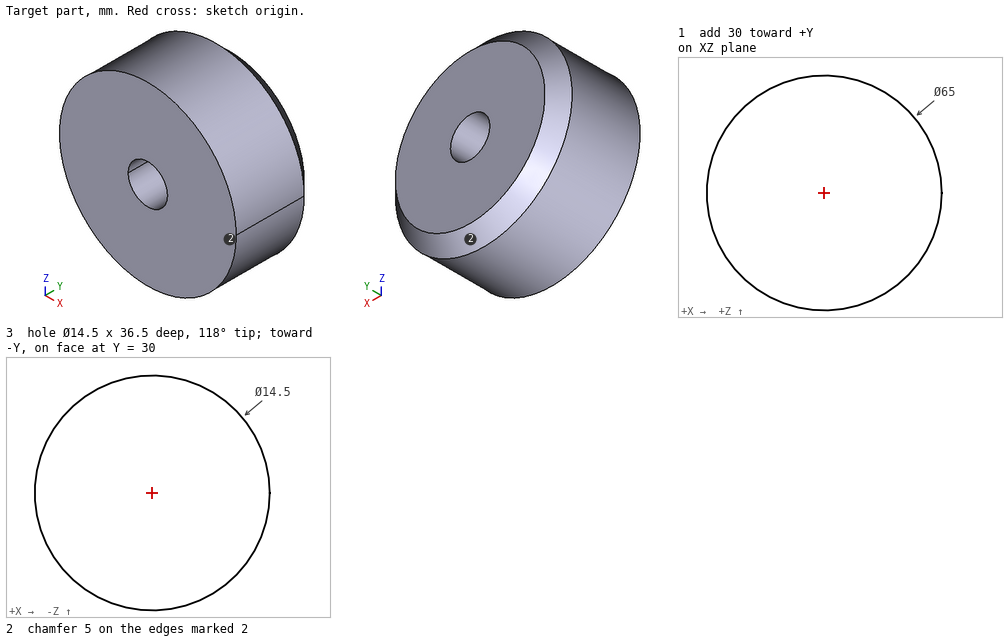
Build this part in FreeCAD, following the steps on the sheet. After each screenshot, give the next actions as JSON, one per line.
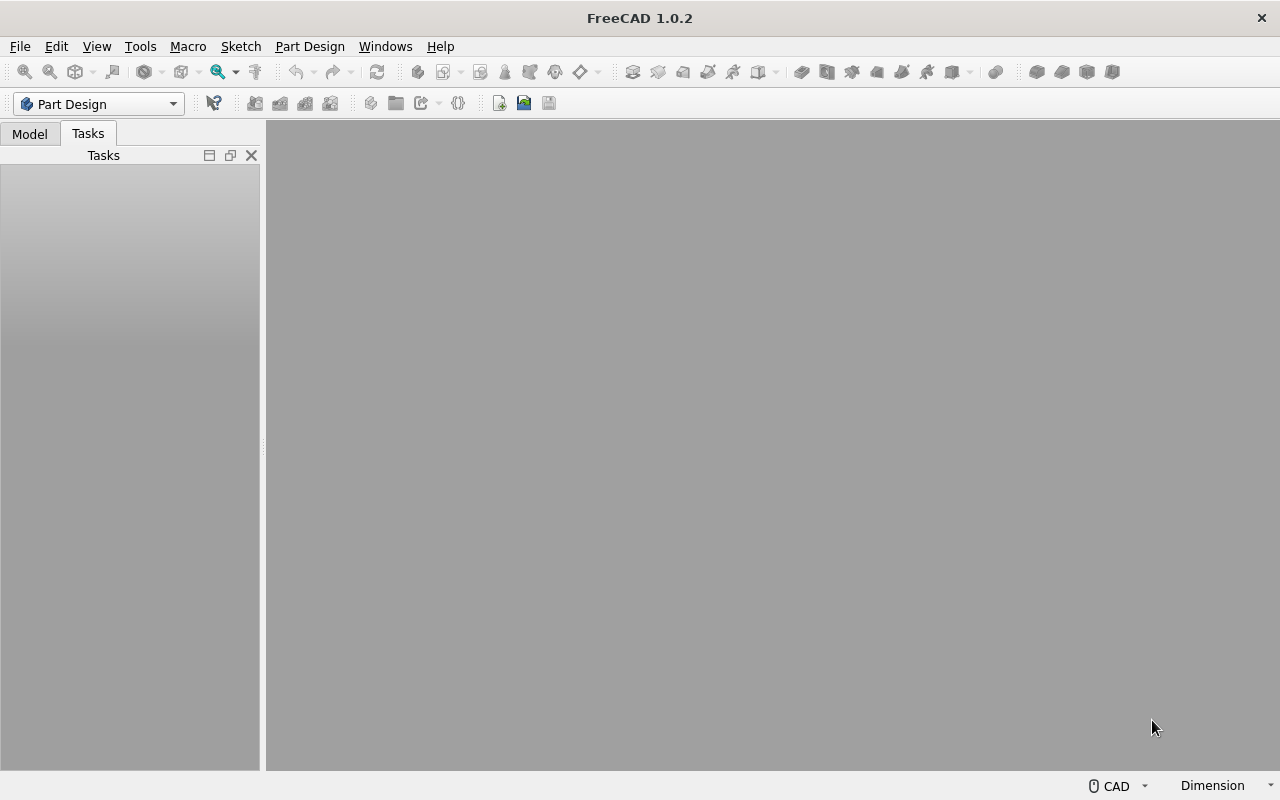
{"action": "left_click", "coordinate": [499, 104]}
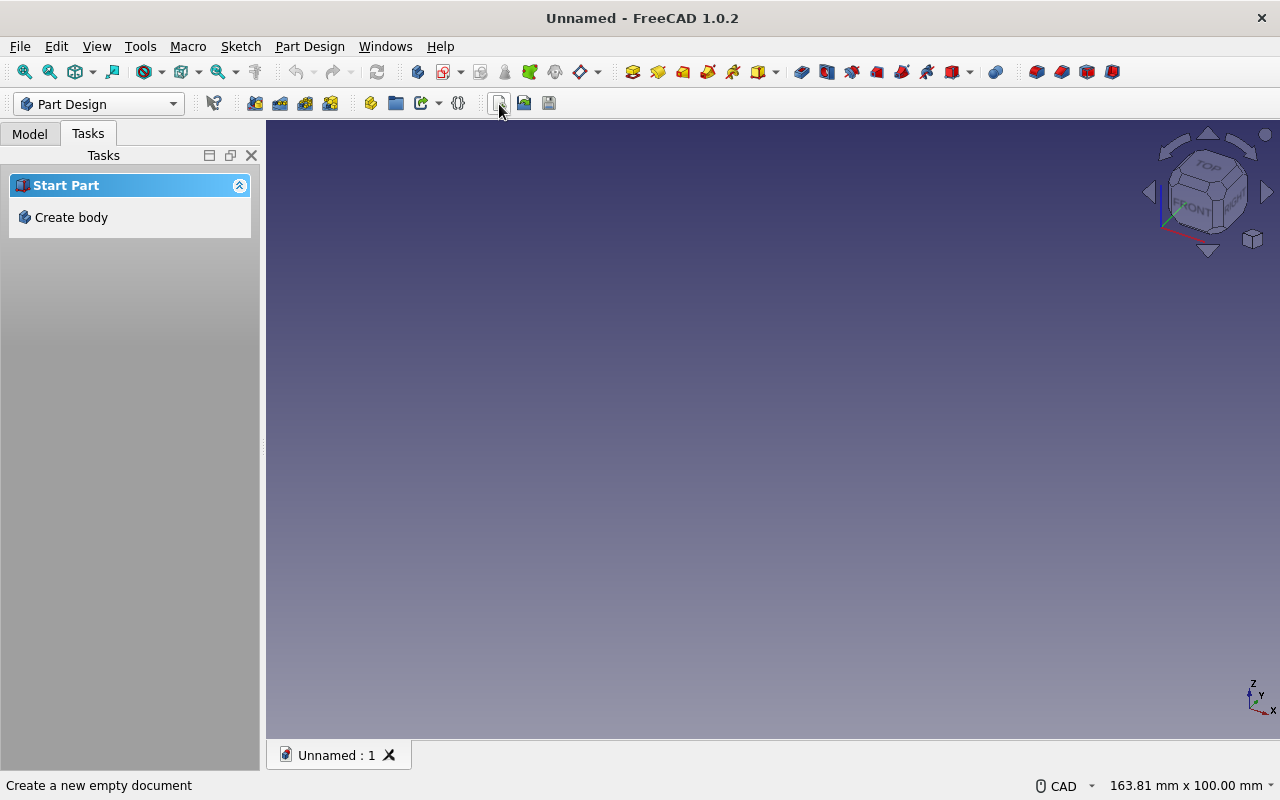
{"action": "left_click", "coordinate": [442, 72]}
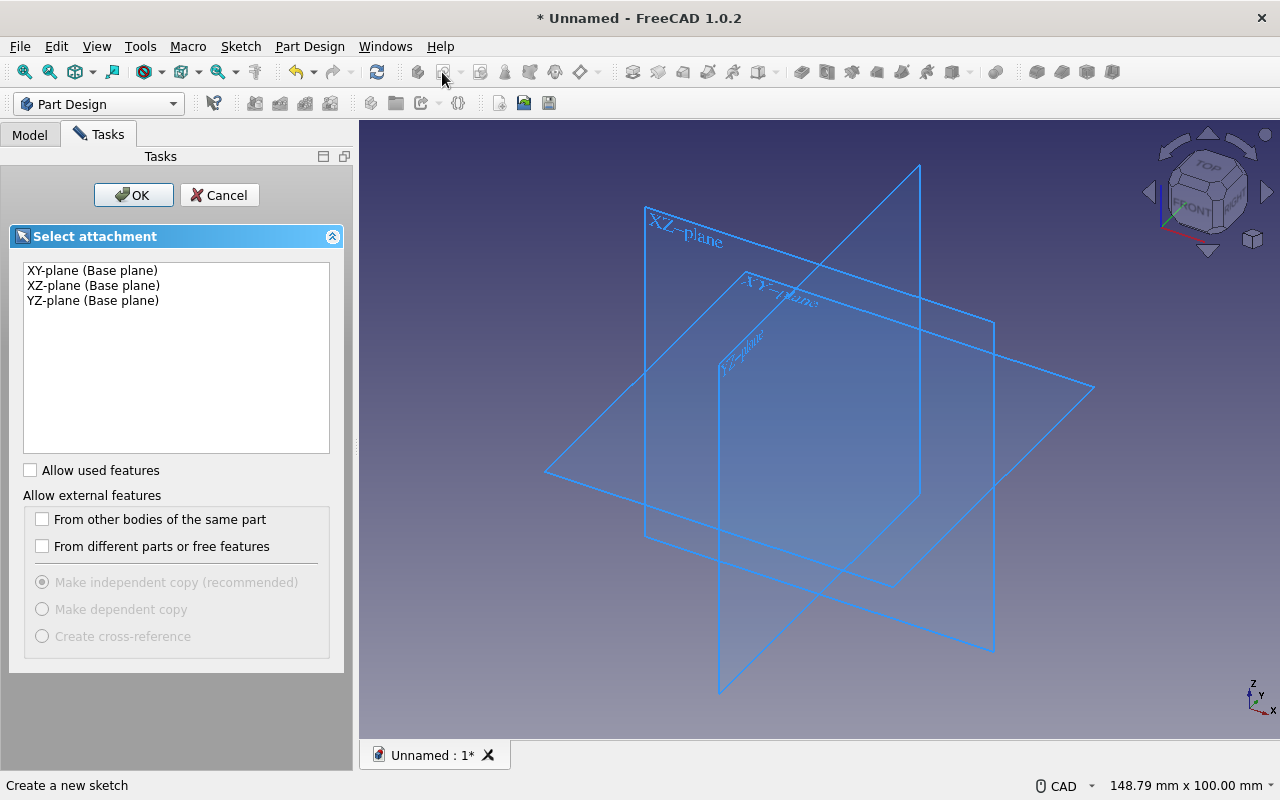
{"action": "left_click", "coordinate": [84, 286]}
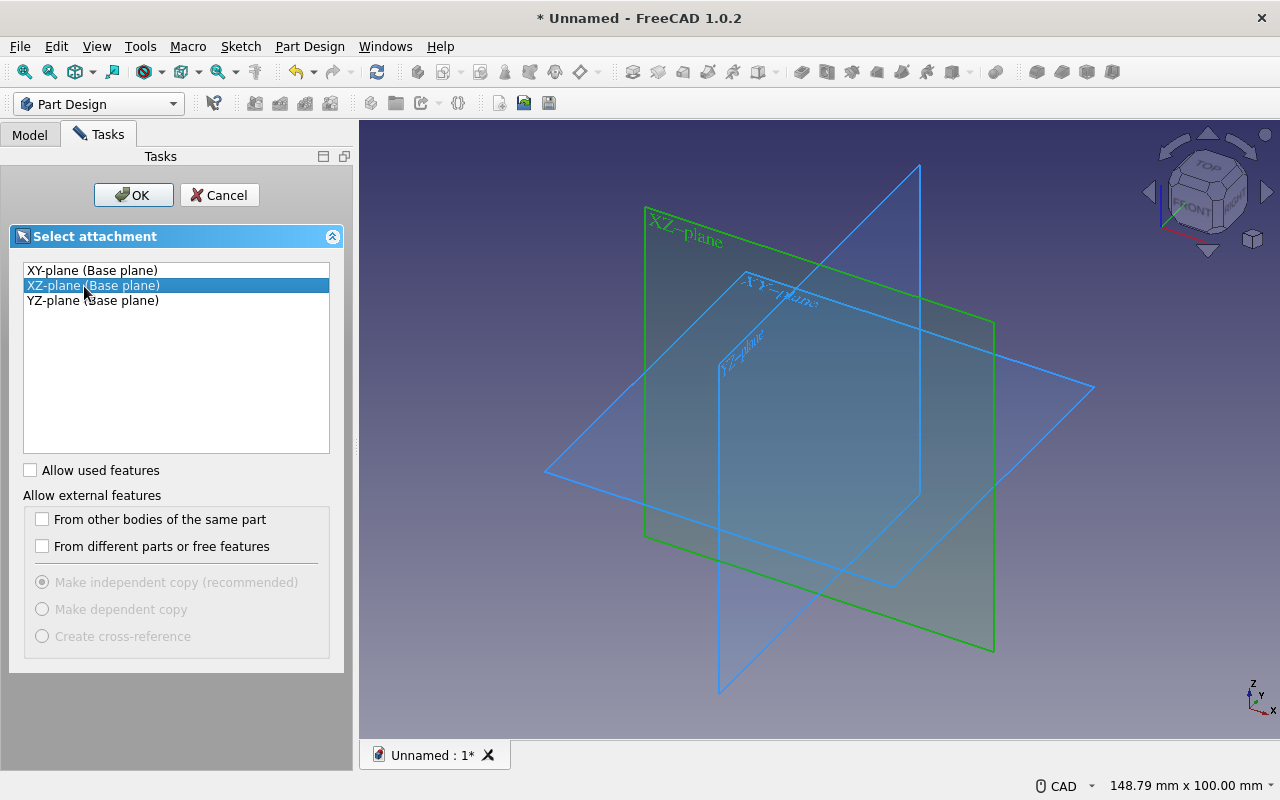
{"action": "left_click", "coordinate": [134, 195]}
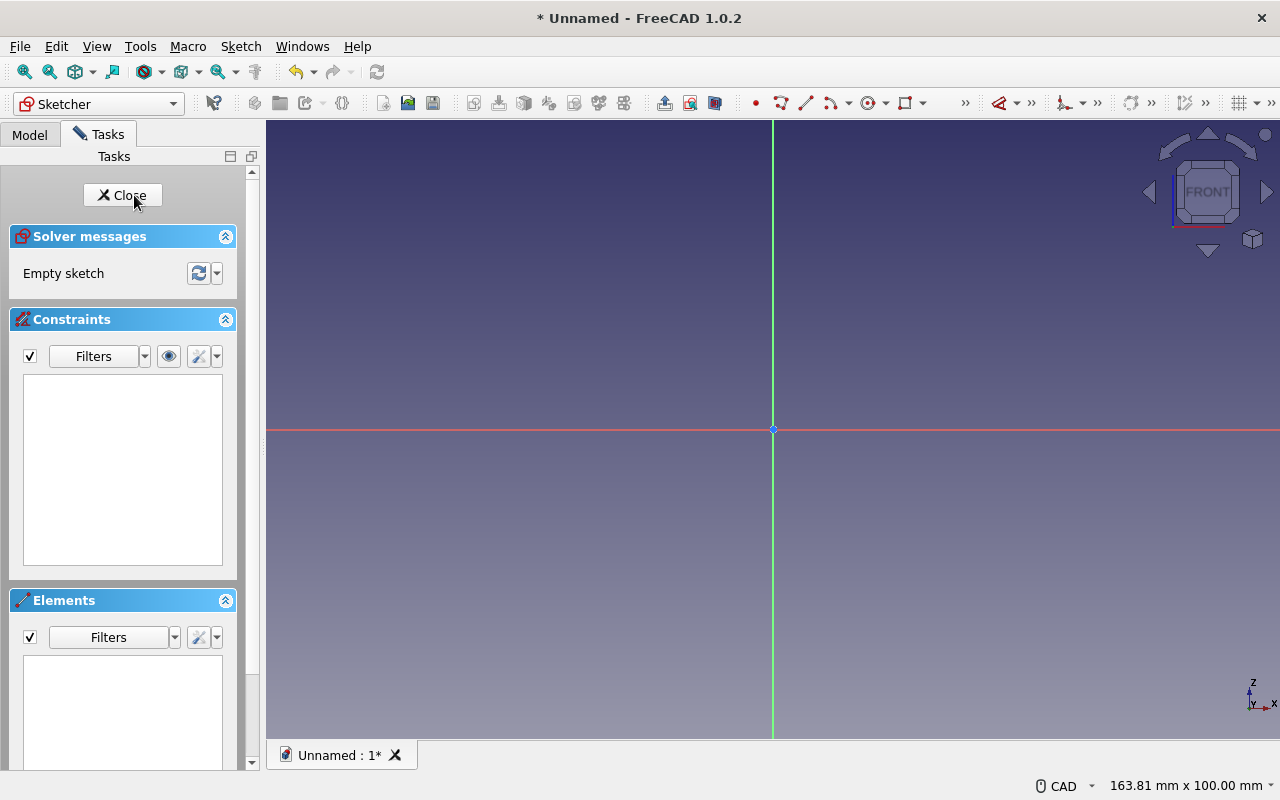
{"action": "left_click", "coordinate": [868, 104]}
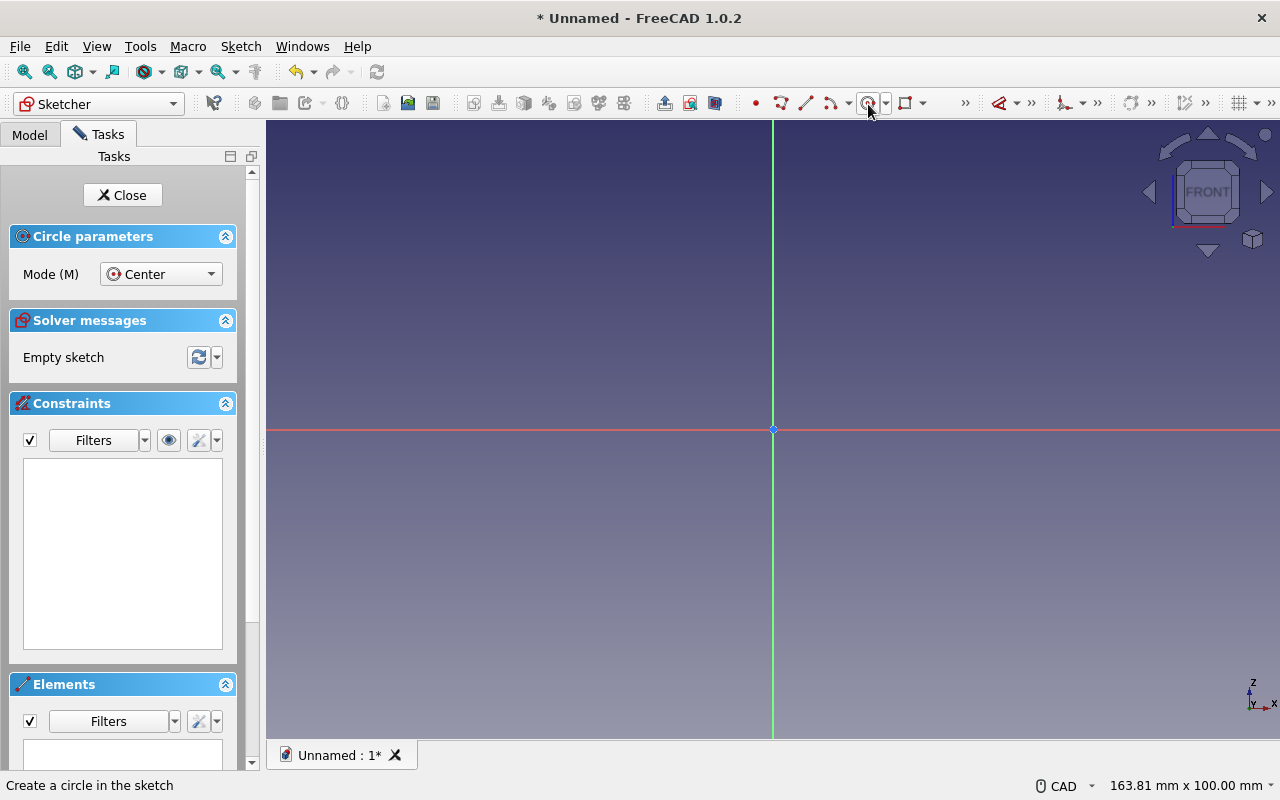
{"action": "left_click", "coordinate": [773, 430]}
{"action": "left_click", "coordinate": [915, 287]}
{"action": "key", "text": "Escape"}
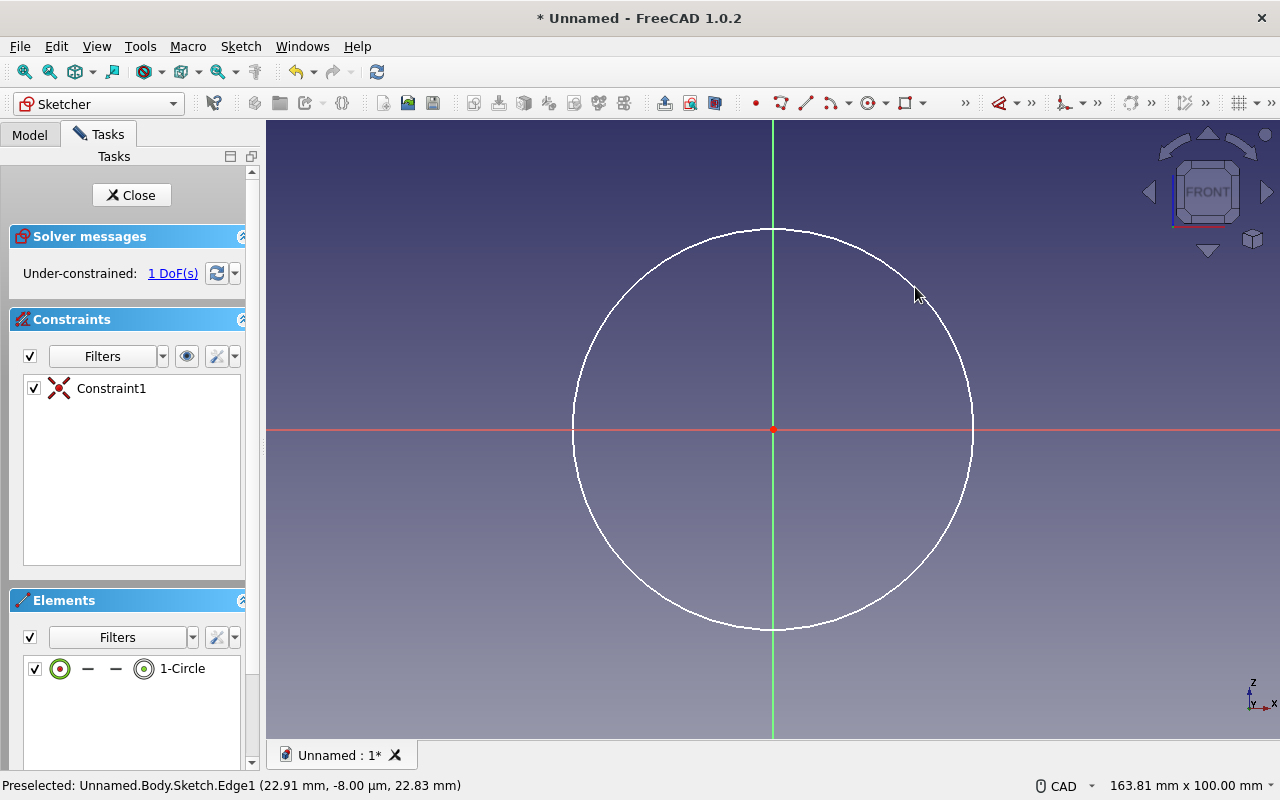
{"action": "left_click", "coordinate": [998, 104]}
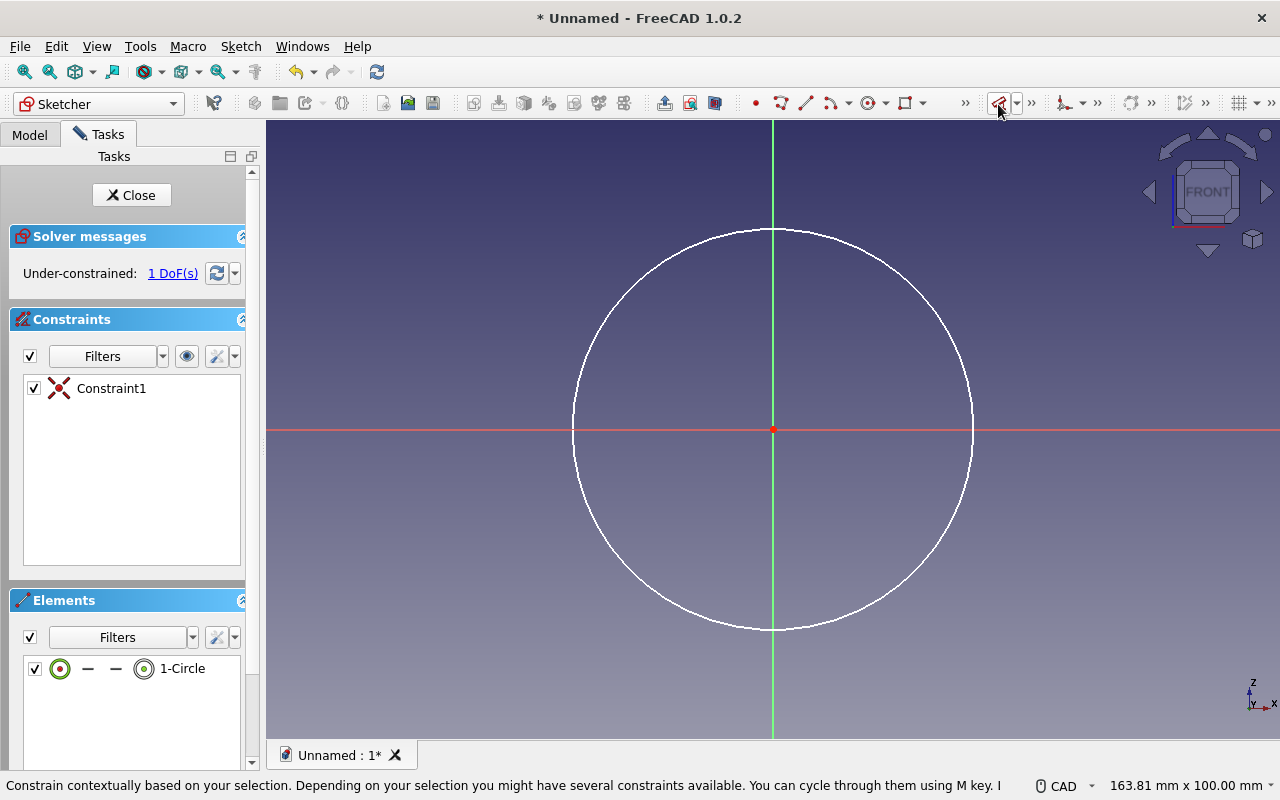
{"action": "left_click", "coordinate": [914, 287]}
{"action": "left_click", "coordinate": [937, 264]}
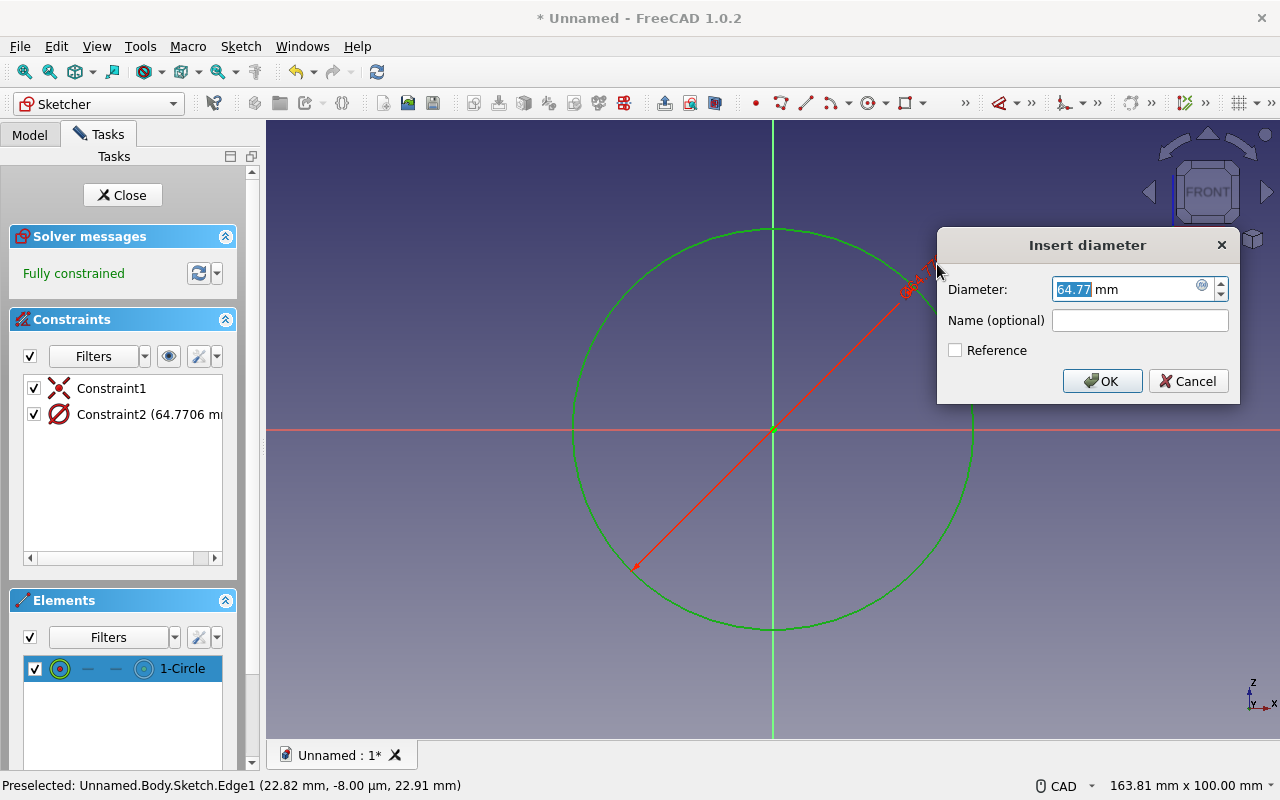
{"action": "type", "text": "65"}
{"action": "key", "text": "Return"}
{"action": "key", "text": "Escape"}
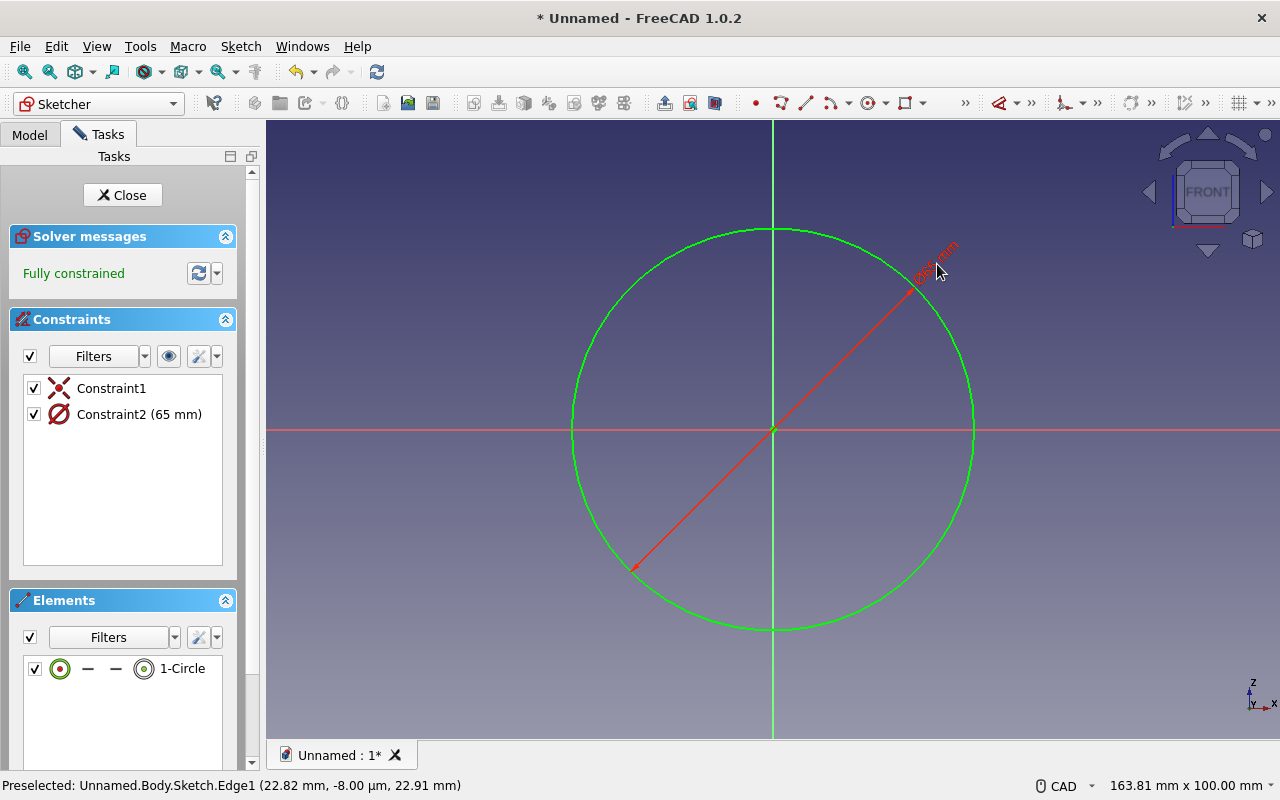
{"action": "left_click", "coordinate": [123, 195]}